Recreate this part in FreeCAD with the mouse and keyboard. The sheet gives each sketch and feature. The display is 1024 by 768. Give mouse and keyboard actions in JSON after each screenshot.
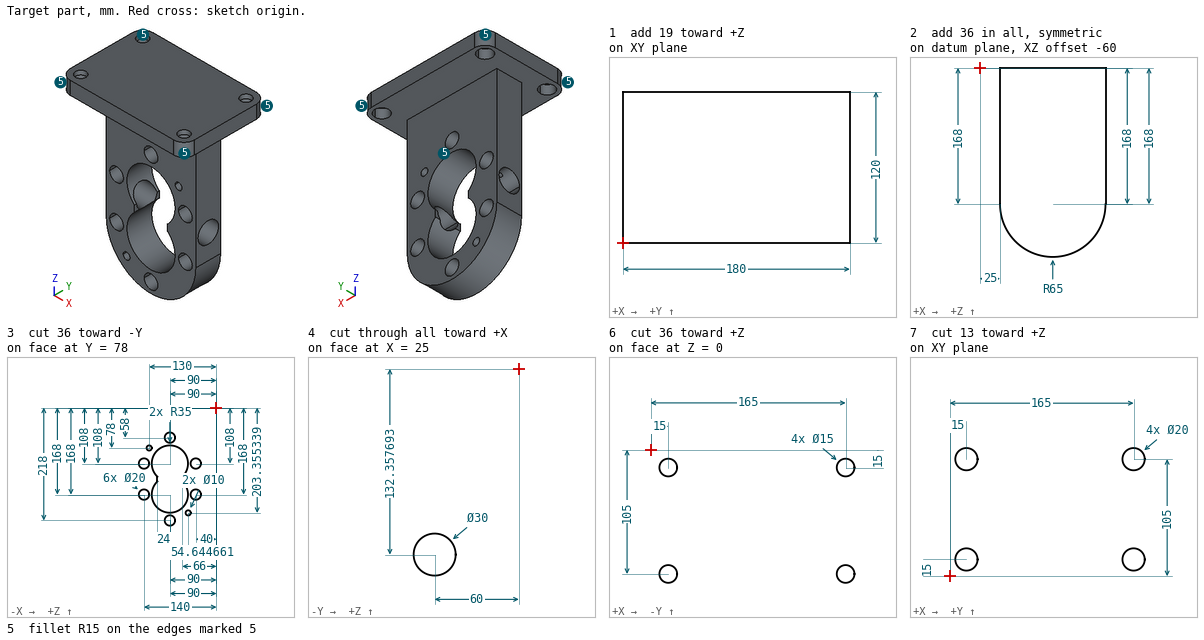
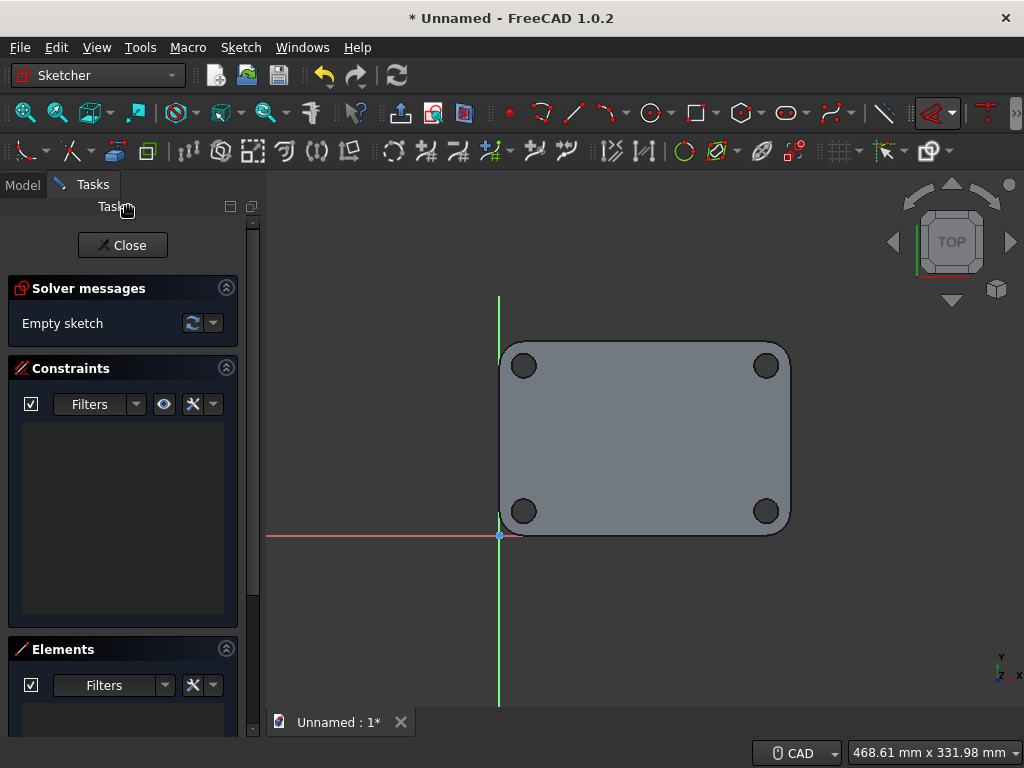
{"action": "left_click", "coordinate": [466, 114]}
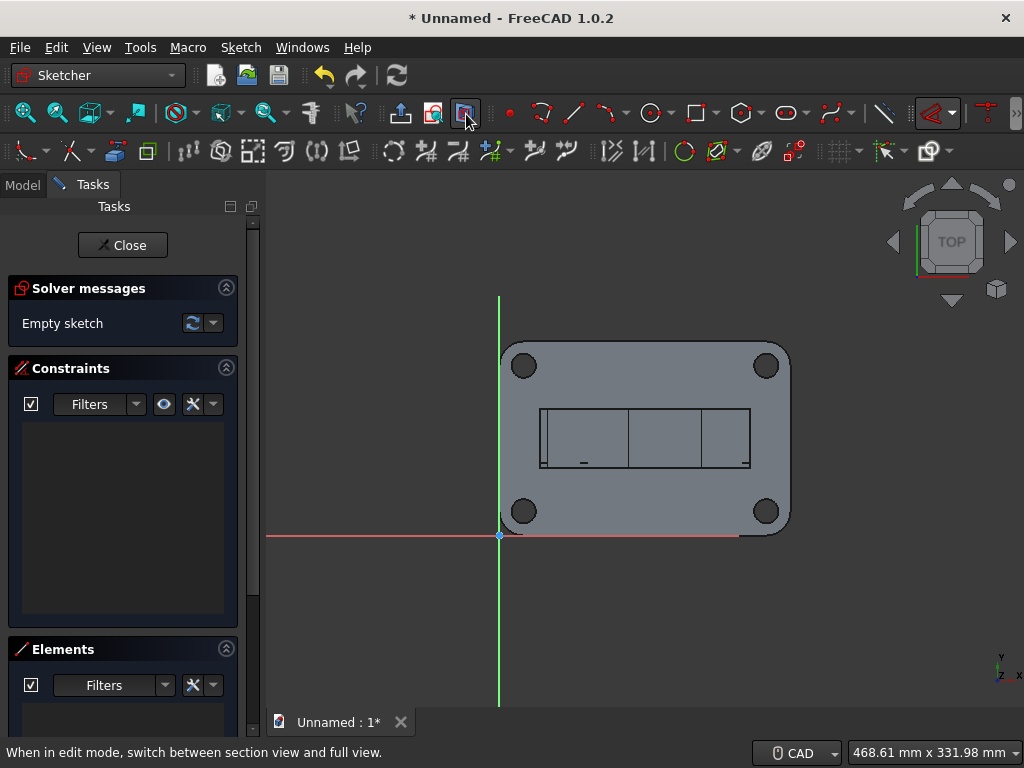
{"action": "scroll", "coordinate": [772, 451], "scroll_direction": "up", "scroll_amount": 2}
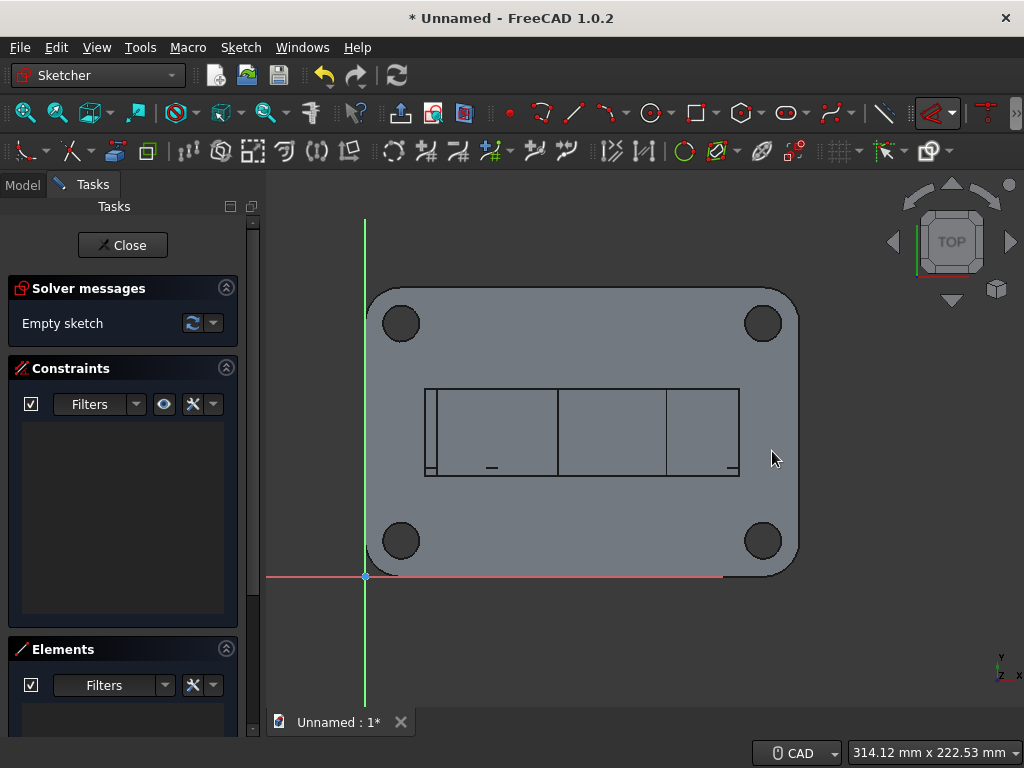
{"action": "left_click", "coordinate": [652, 114]}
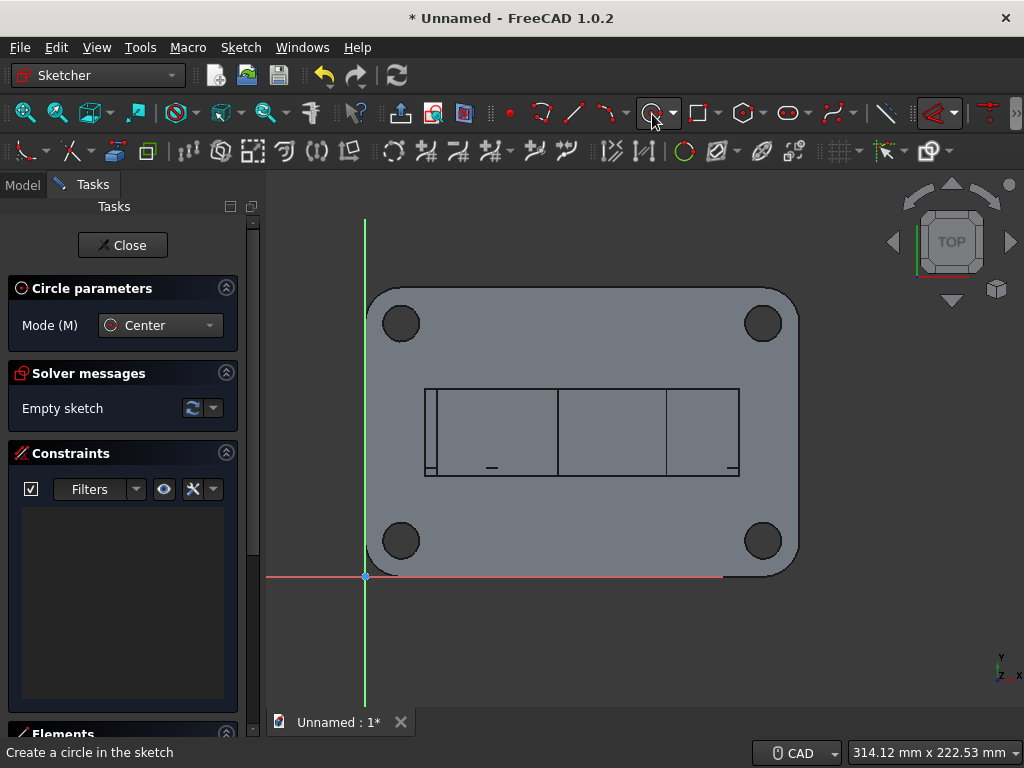
{"action": "left_click", "coordinate": [763, 324]}
{"action": "left_click", "coordinate": [780, 306]}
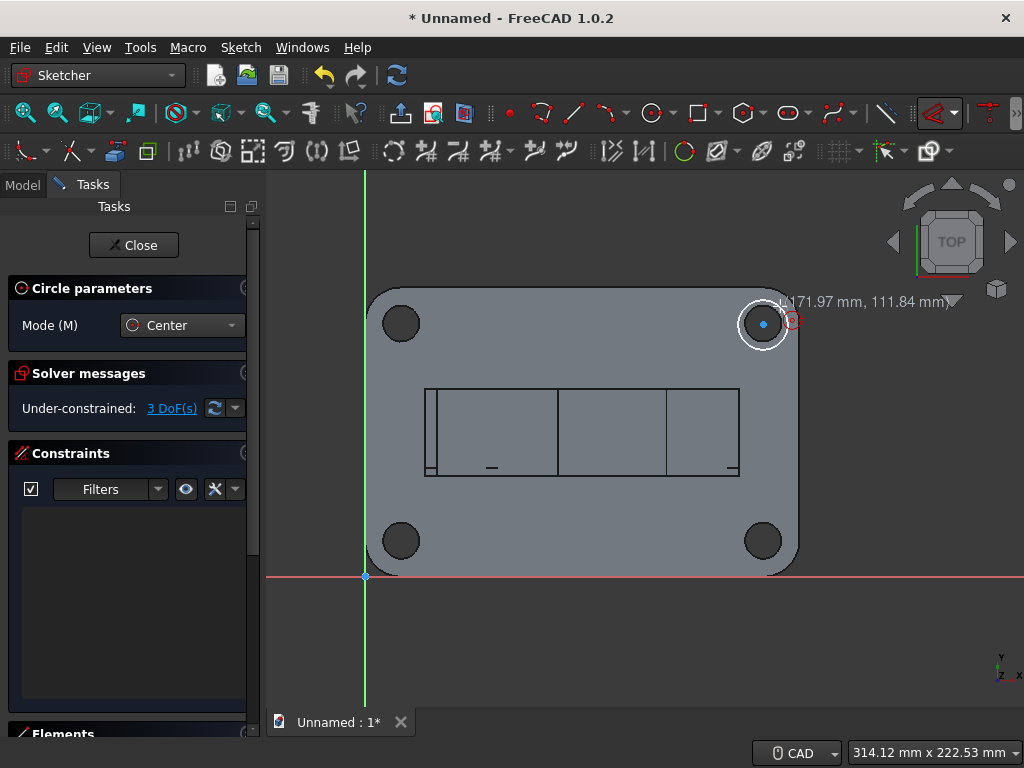
{"action": "left_click", "coordinate": [401, 324]}
{"action": "left_click", "coordinate": [418, 306]}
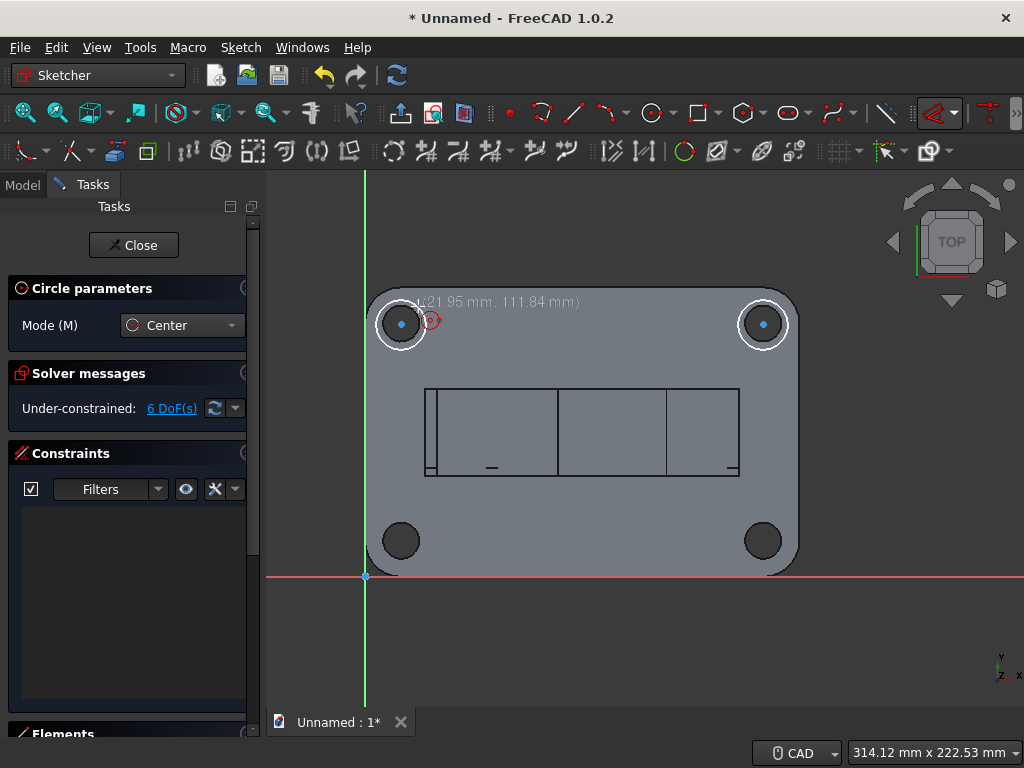
{"action": "left_click", "coordinate": [401, 541]}
{"action": "left_click", "coordinate": [418, 524]}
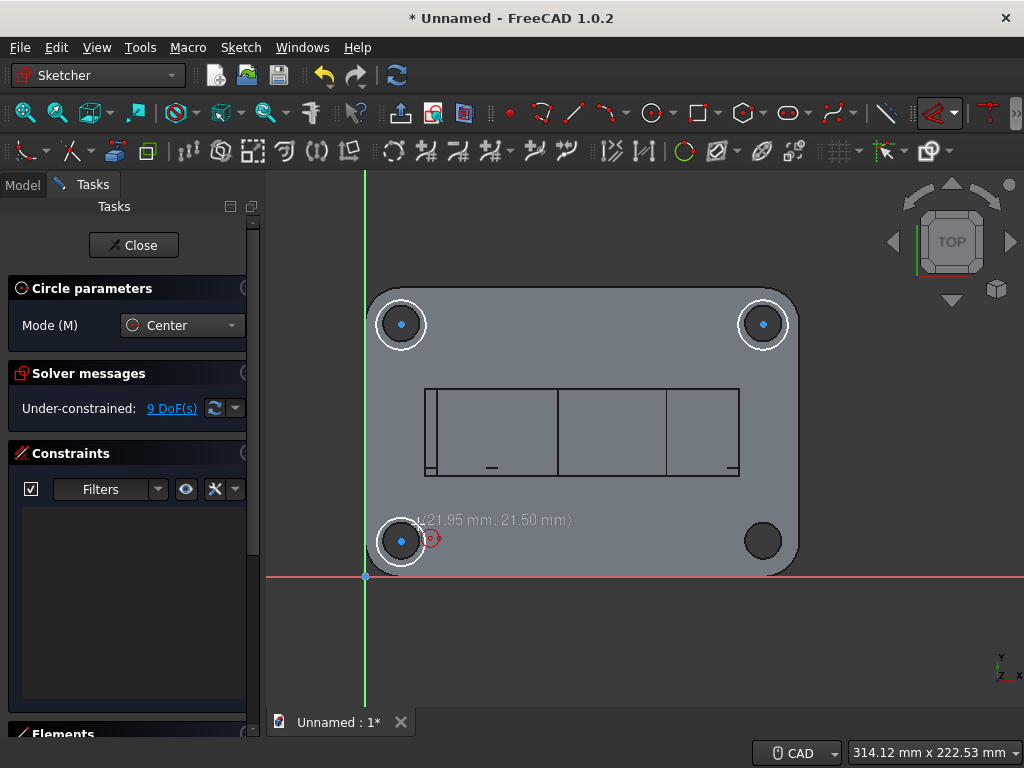
{"action": "left_click", "coordinate": [763, 541]}
{"action": "left_click", "coordinate": [780, 524]}
{"action": "key", "text": "Escape"}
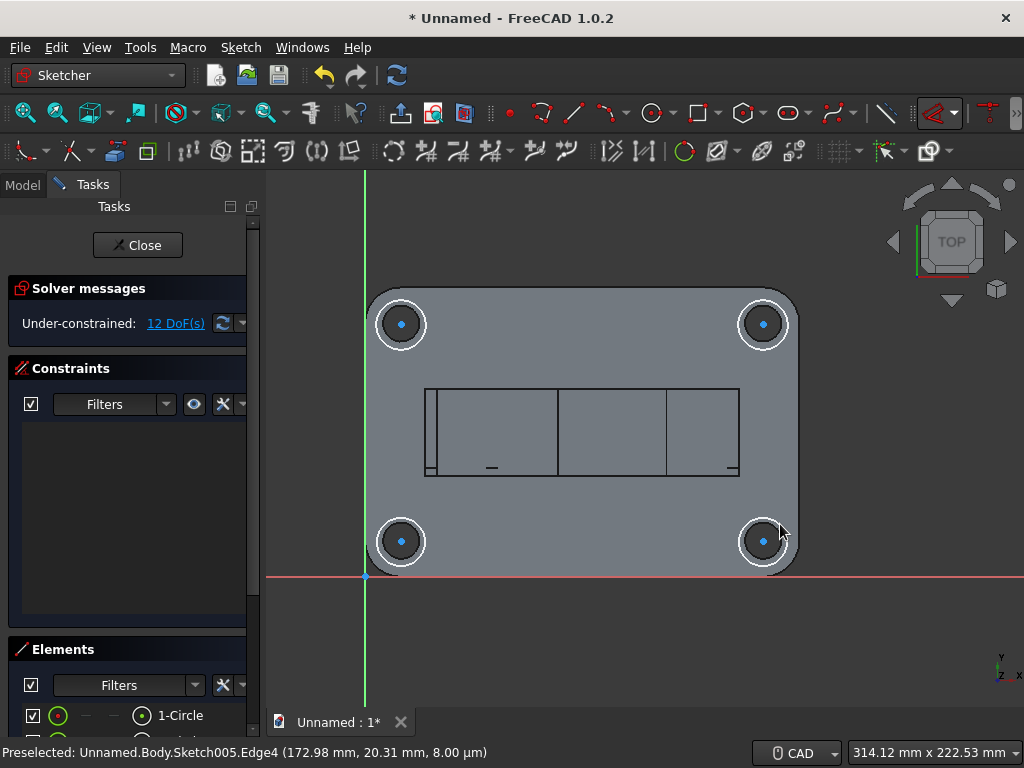
{"action": "left_click", "coordinate": [780, 307]}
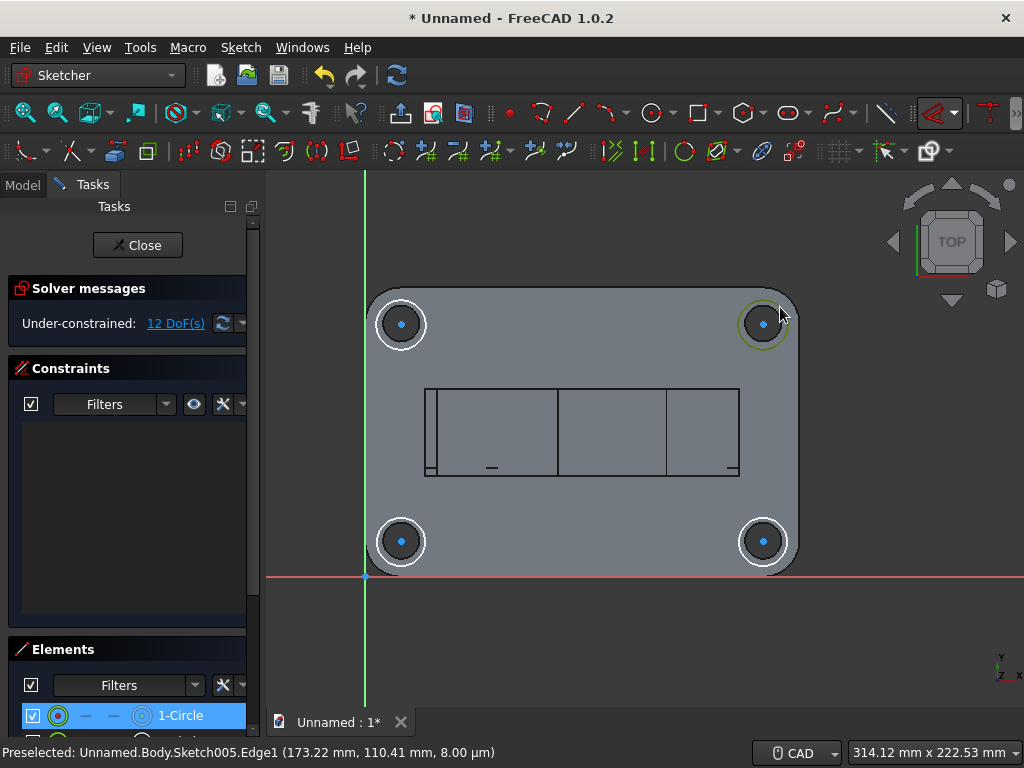
{"action": "left_click", "coordinate": [418, 307]}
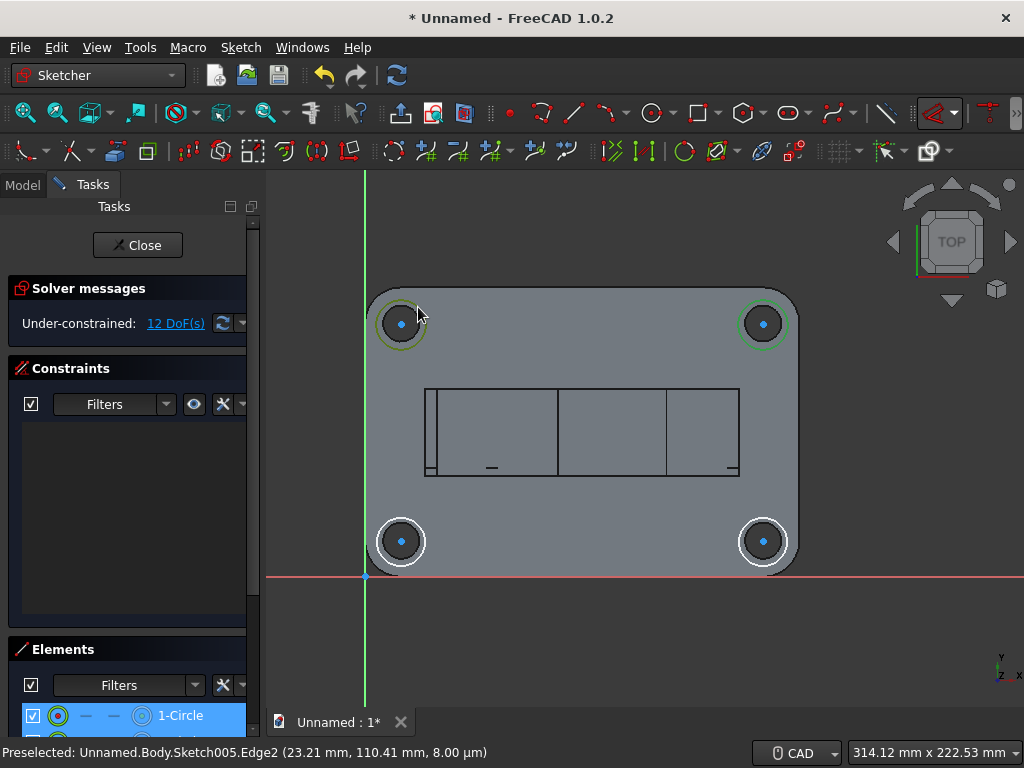
{"action": "left_click", "coordinate": [418, 525]}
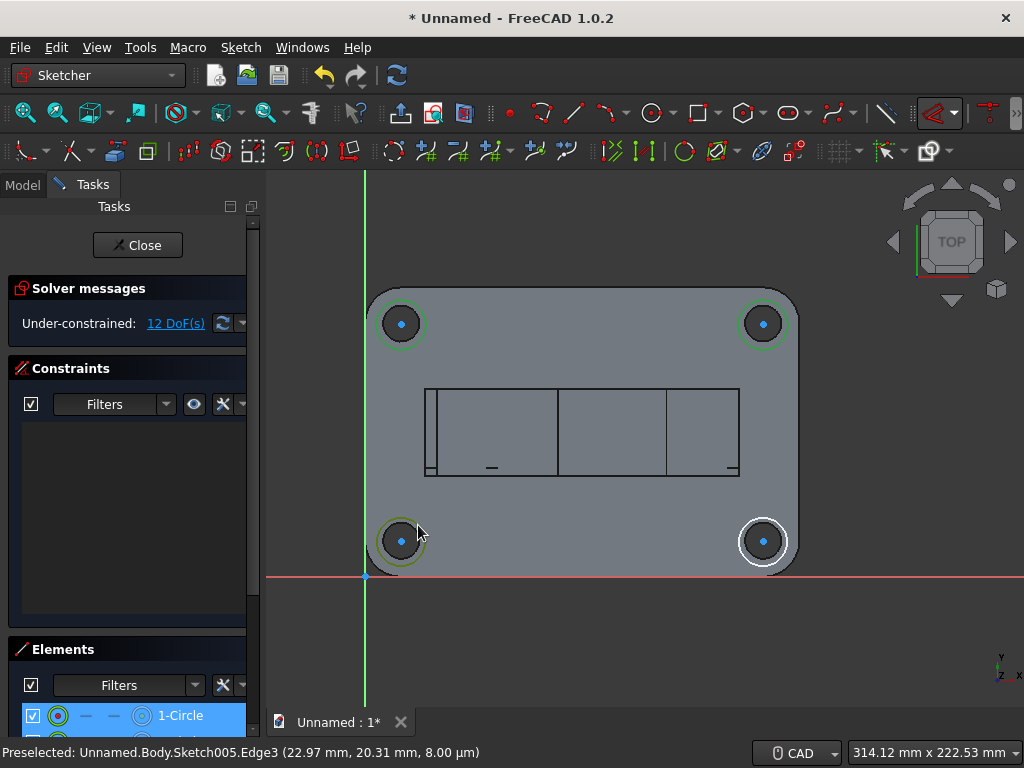
{"action": "left_click", "coordinate": [780, 525]}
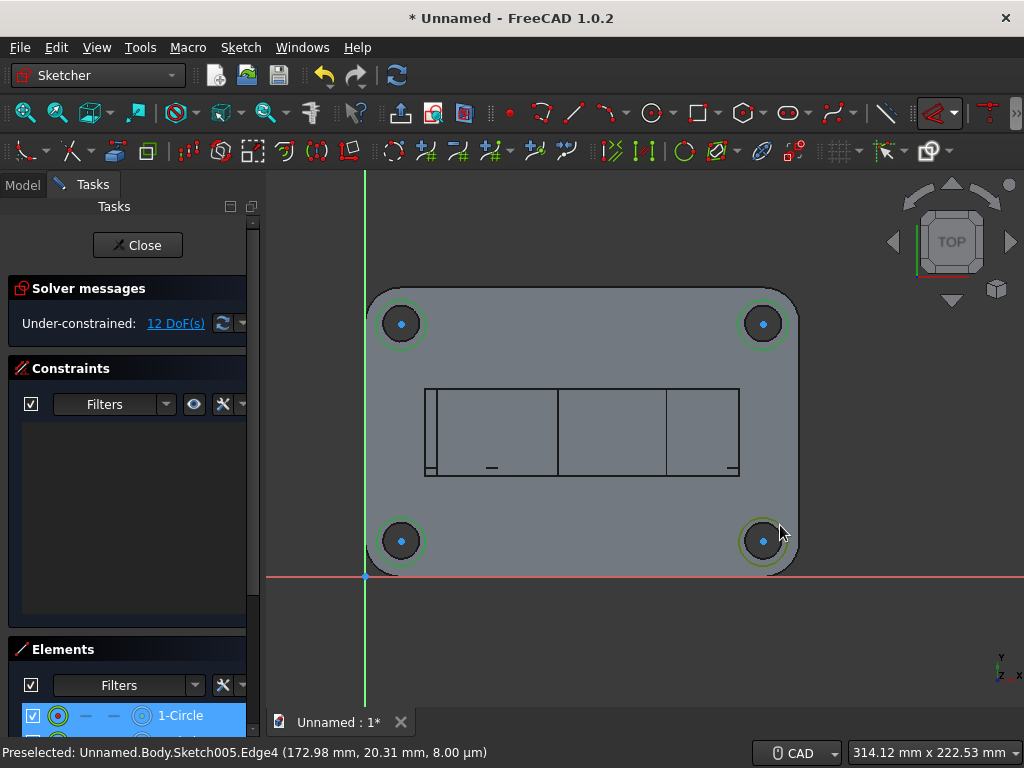
{"action": "key", "text": "e"}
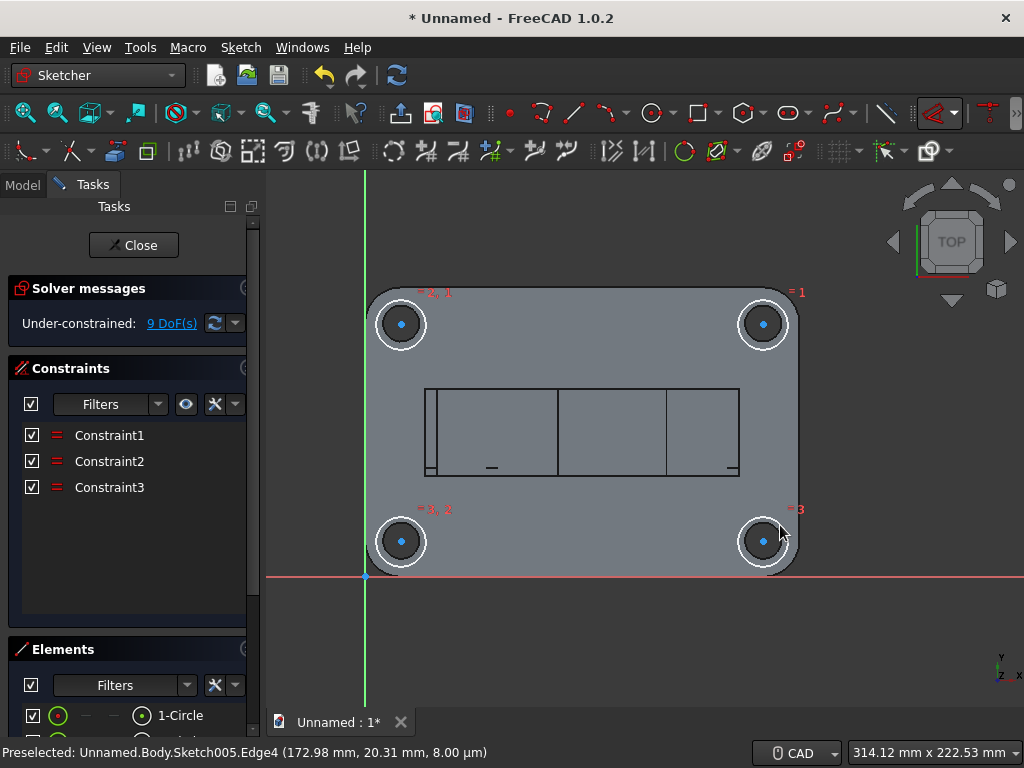
{"action": "left_click", "coordinate": [763, 325]}